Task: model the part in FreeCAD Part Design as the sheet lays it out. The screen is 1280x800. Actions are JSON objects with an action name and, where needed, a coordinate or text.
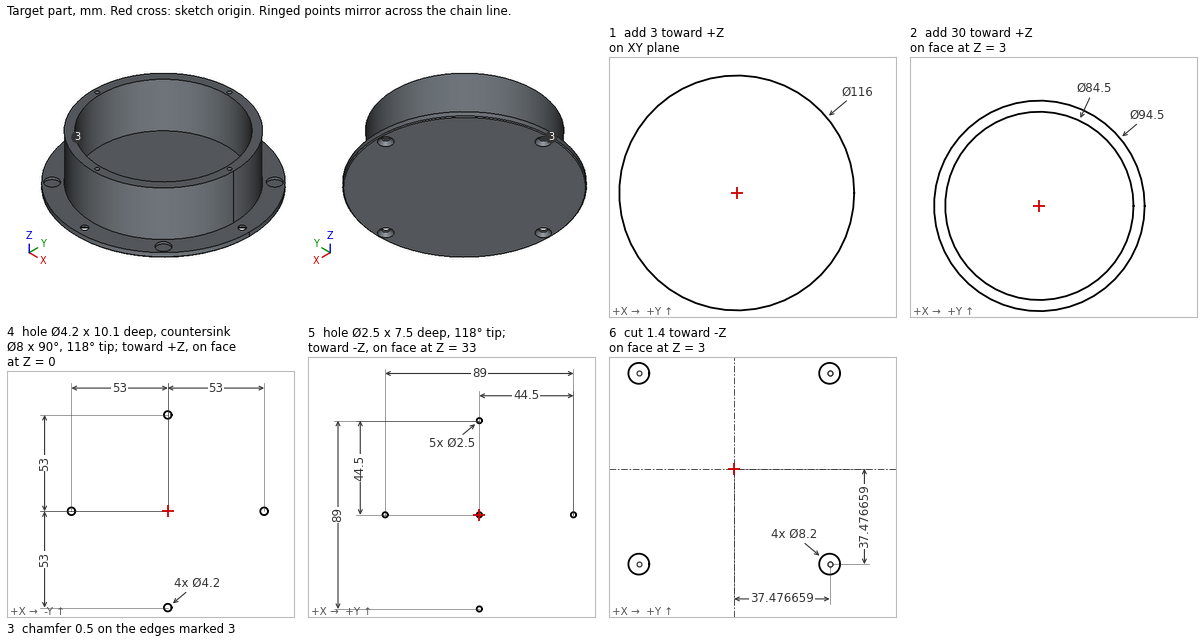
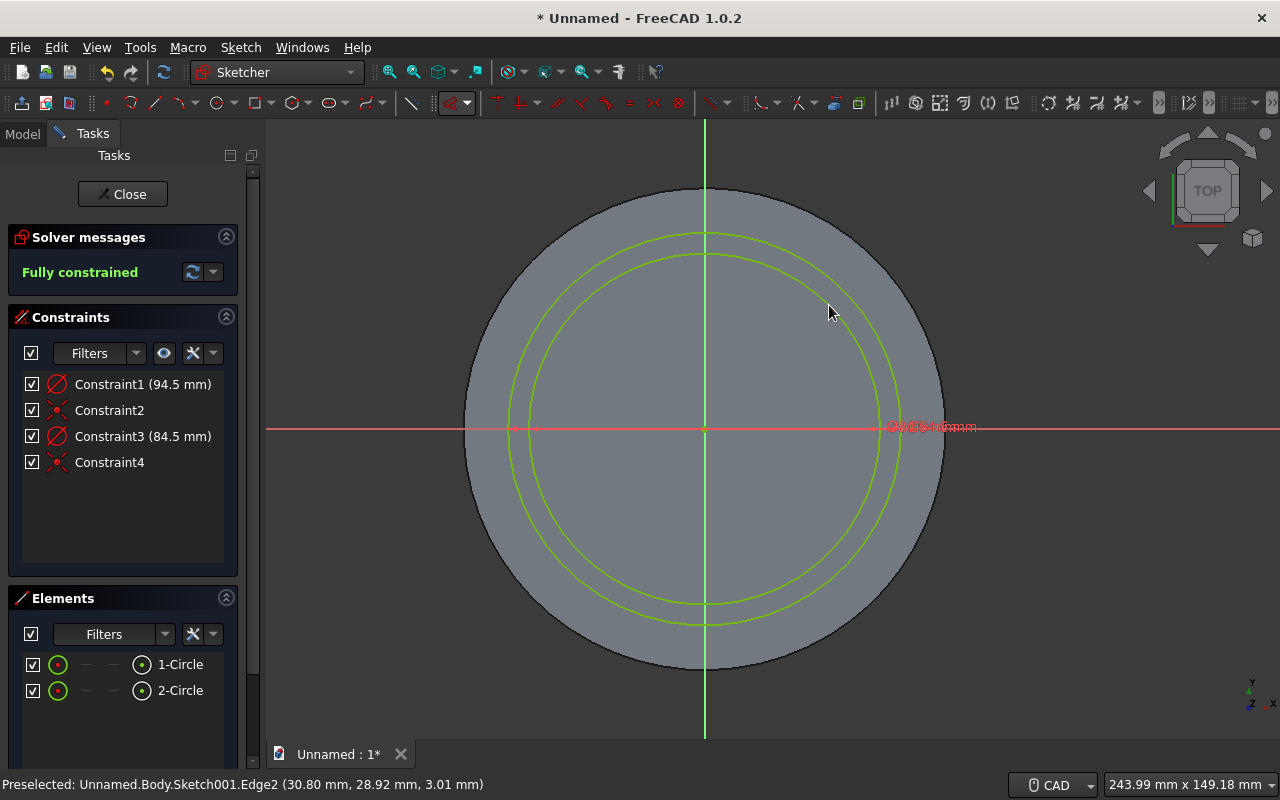
{"action": "left_click", "coordinate": [123, 194]}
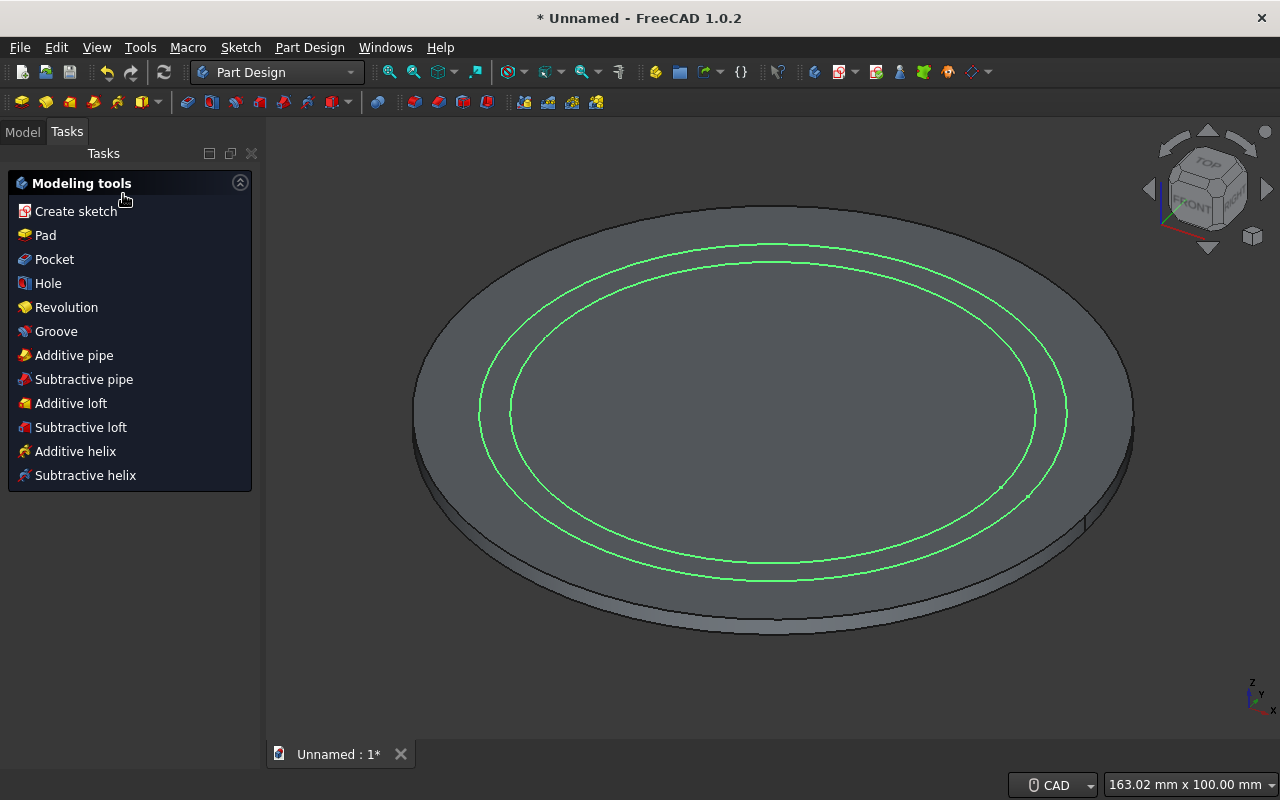
{"action": "left_click", "coordinate": [22, 102]}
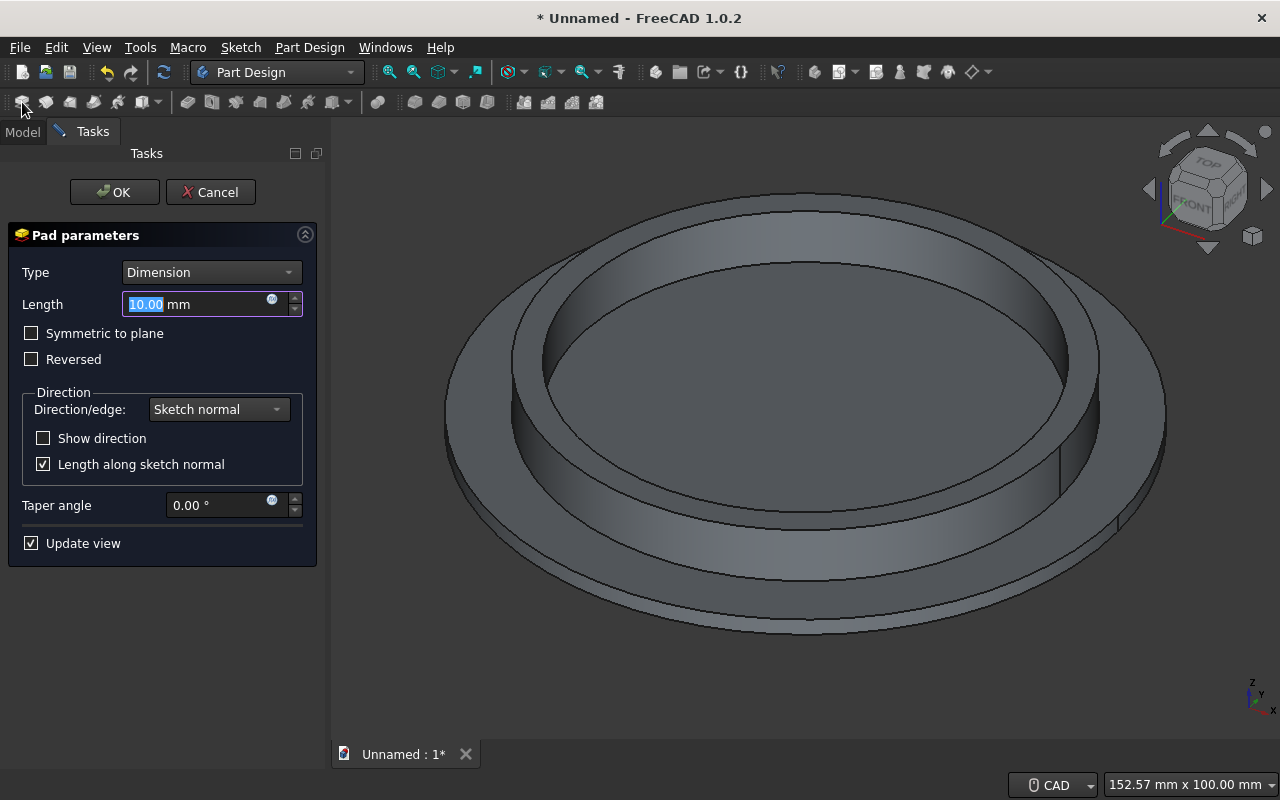
{"action": "type", "text": "30"}
{"action": "key", "text": "Tab"}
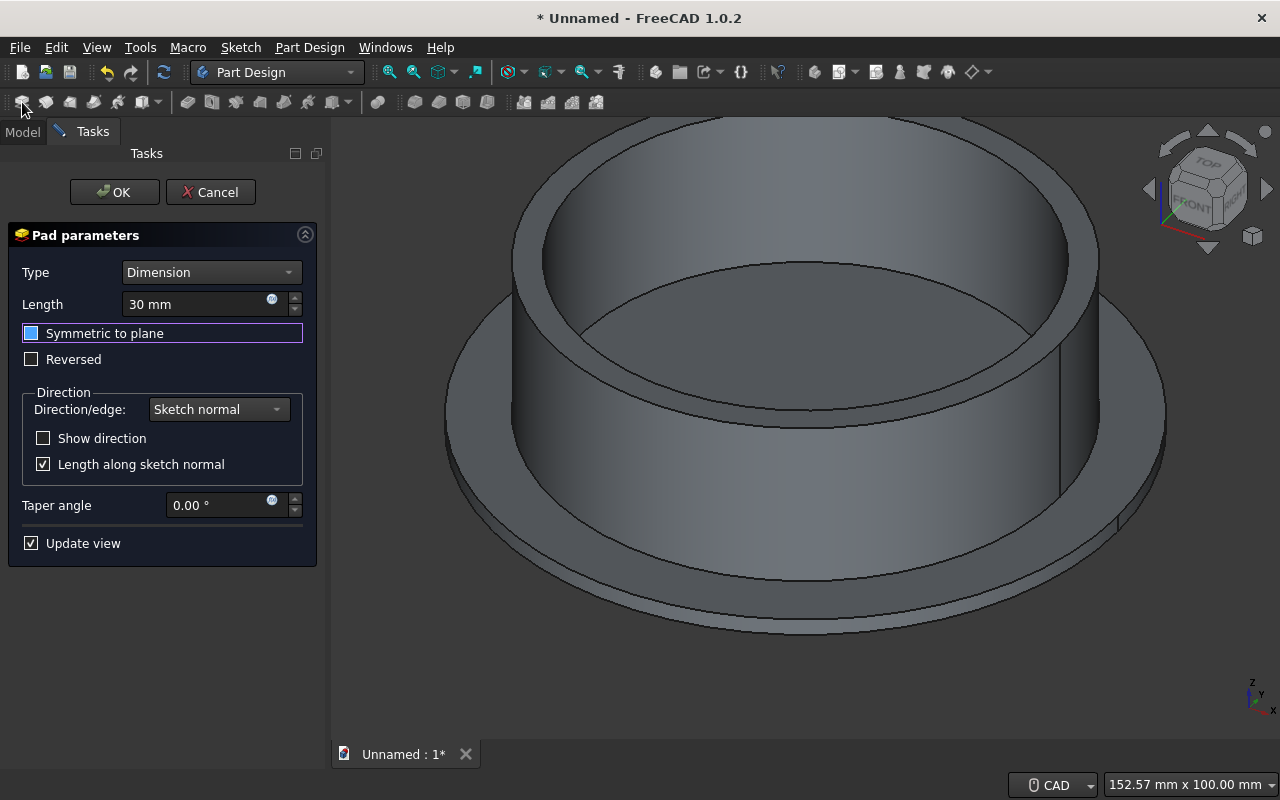
{"action": "left_click", "coordinate": [115, 192]}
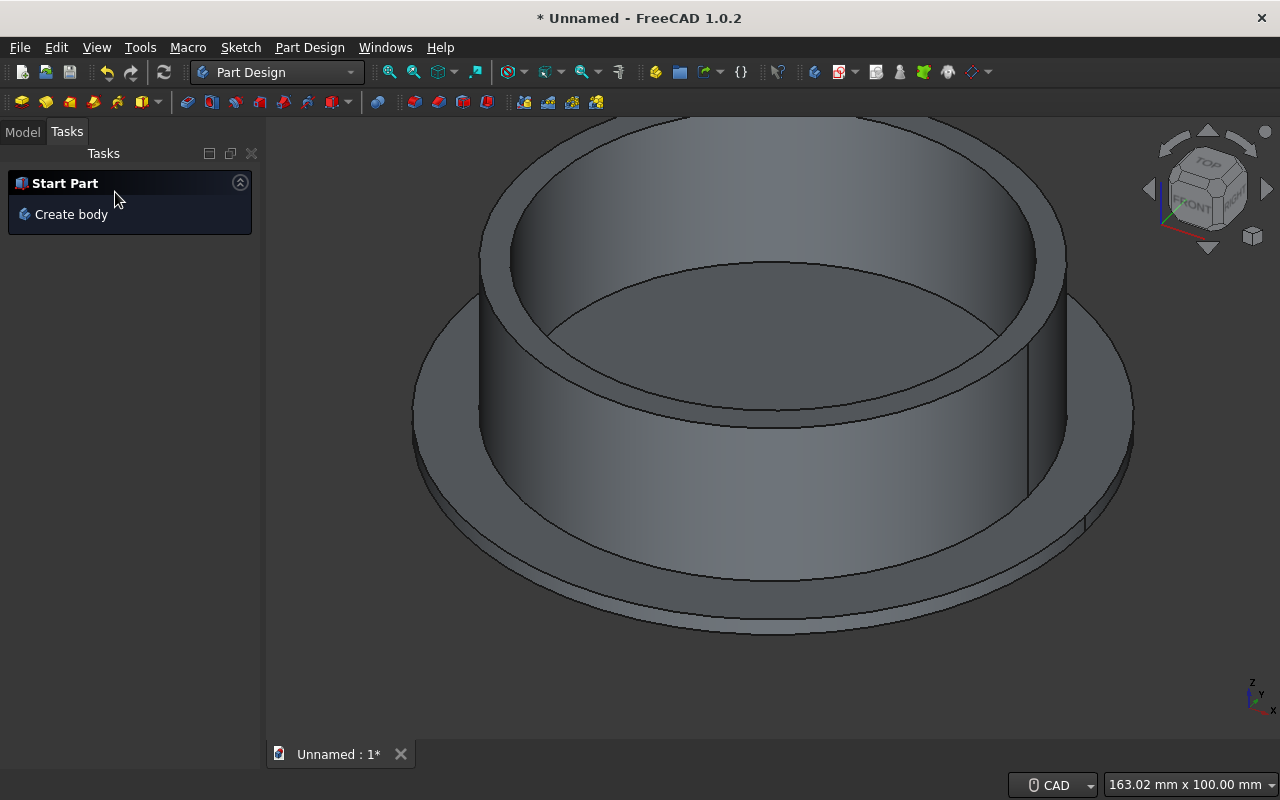
{"action": "left_click", "coordinate": [390, 72]}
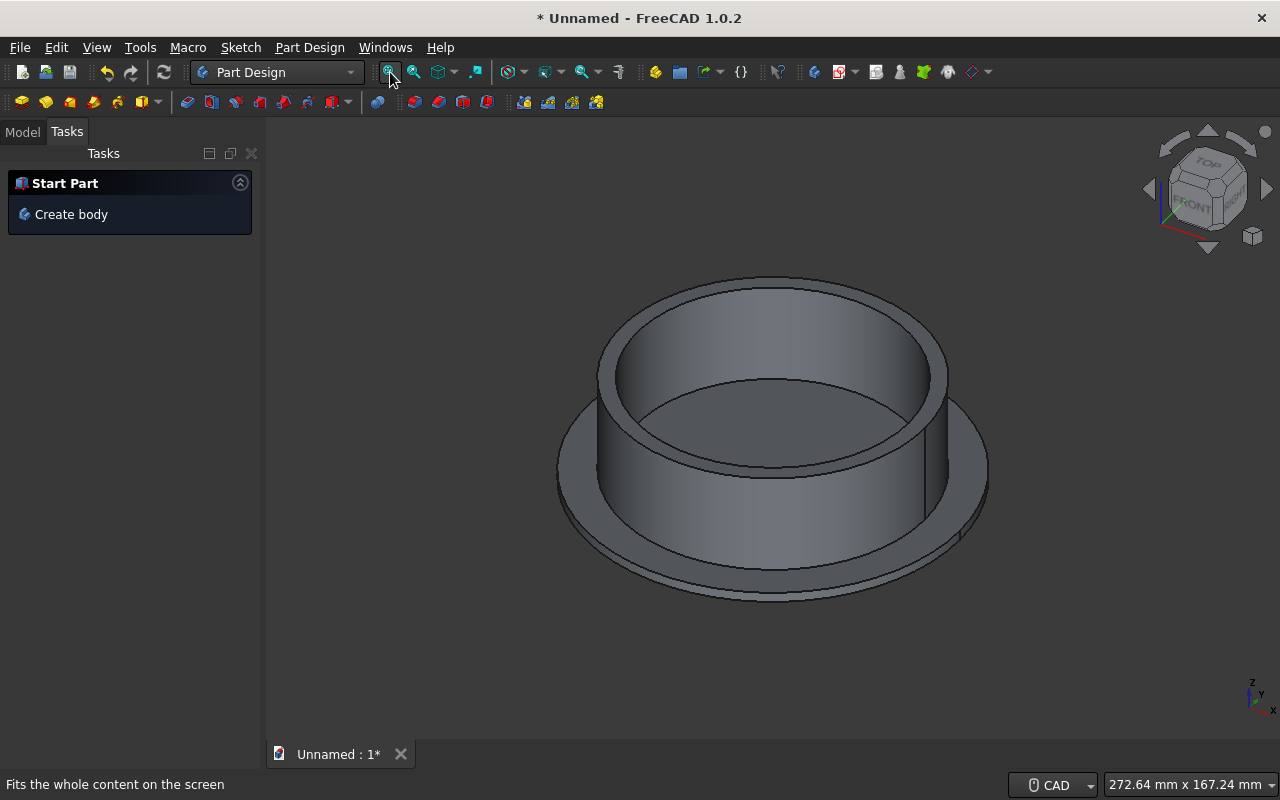
{"action": "left_click", "coordinate": [835, 596]}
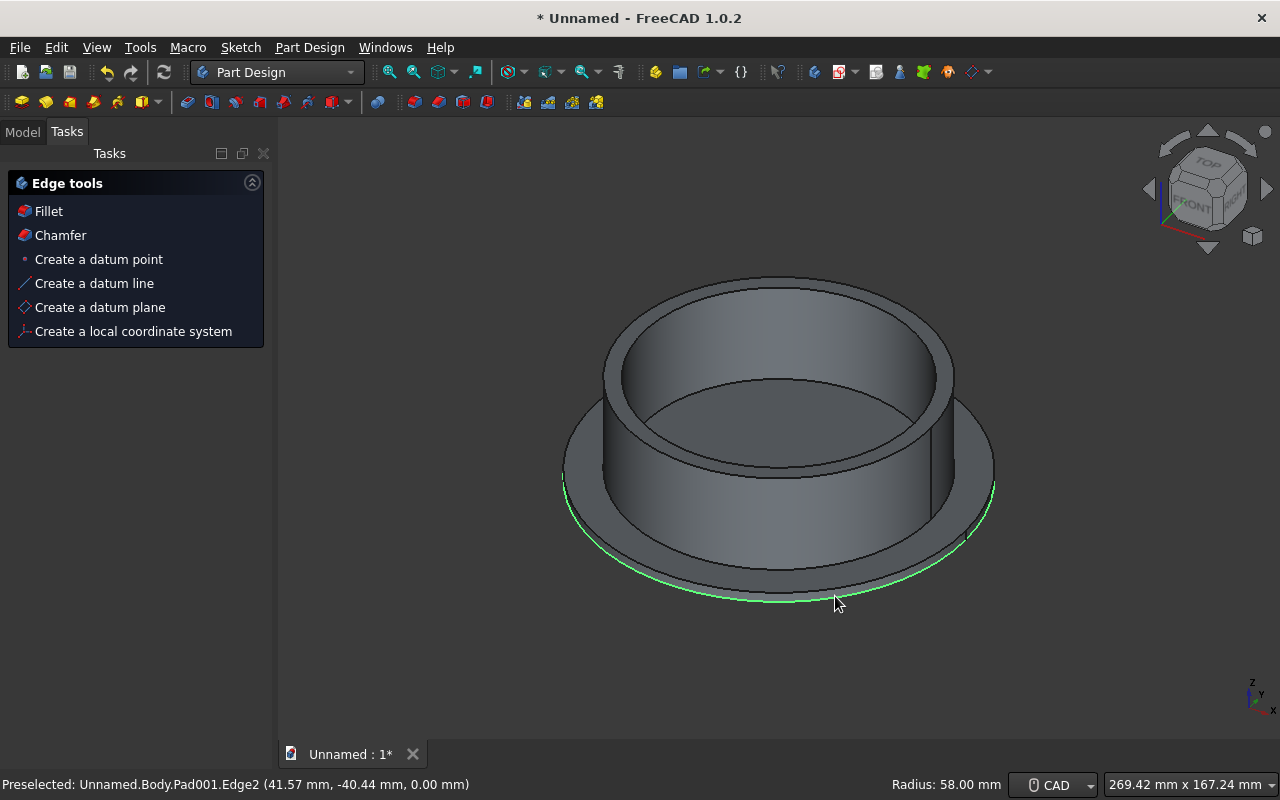
{"action": "left_click", "coordinate": [440, 102]}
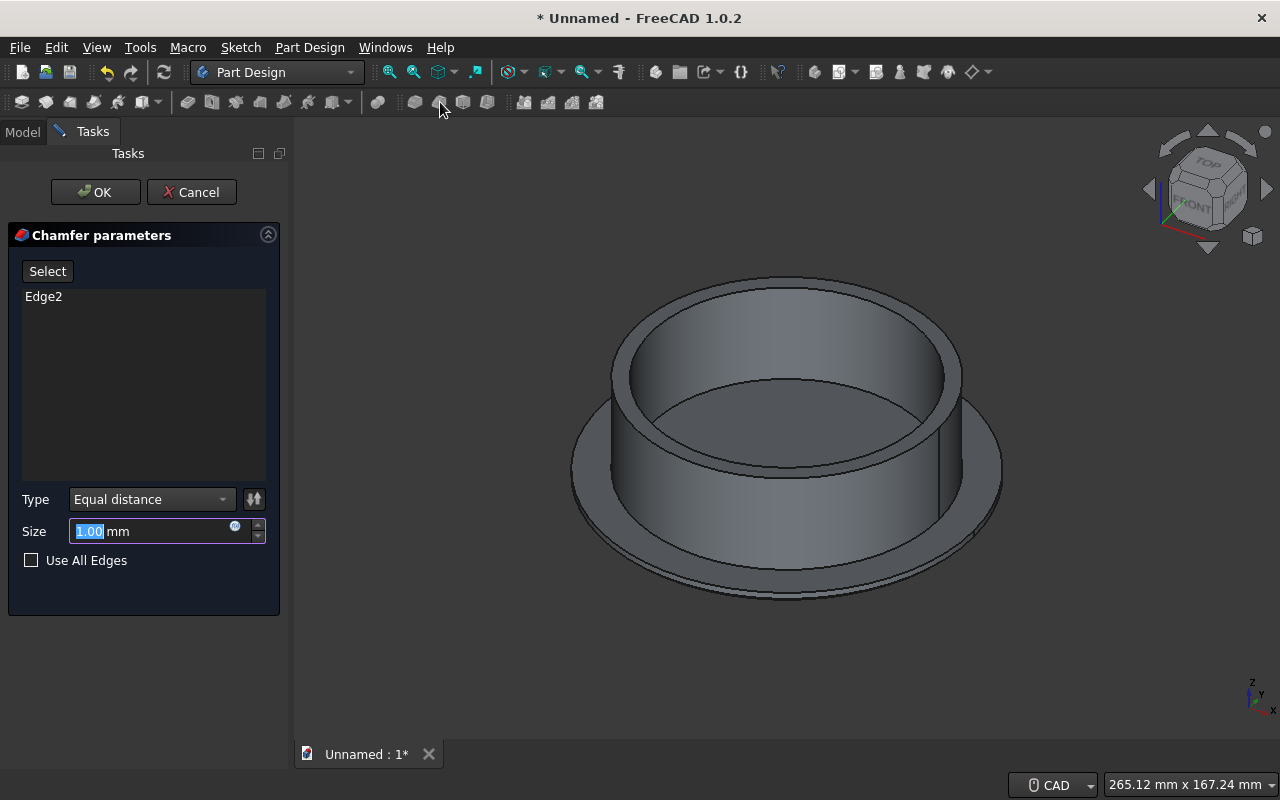
{"action": "type", "text": "0.5"}
{"action": "key", "text": "Tab"}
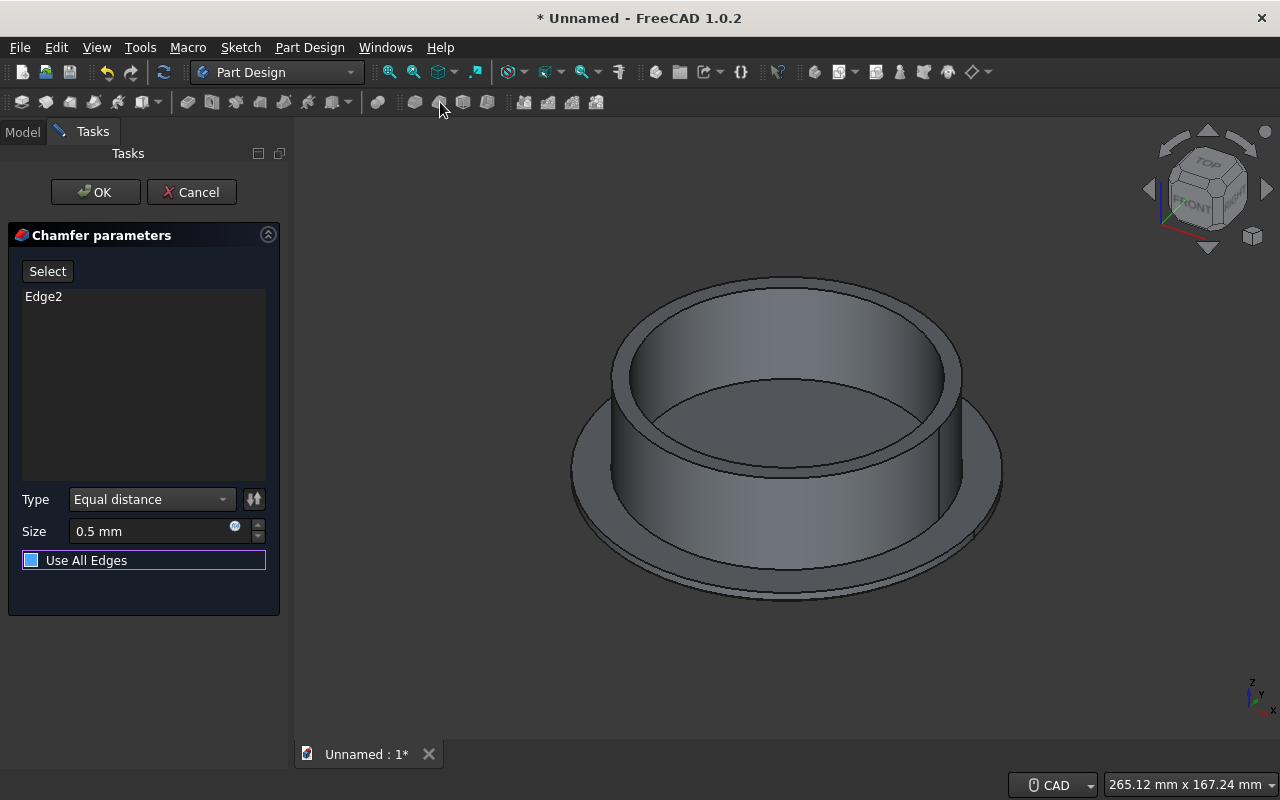
{"action": "left_click", "coordinate": [96, 192]}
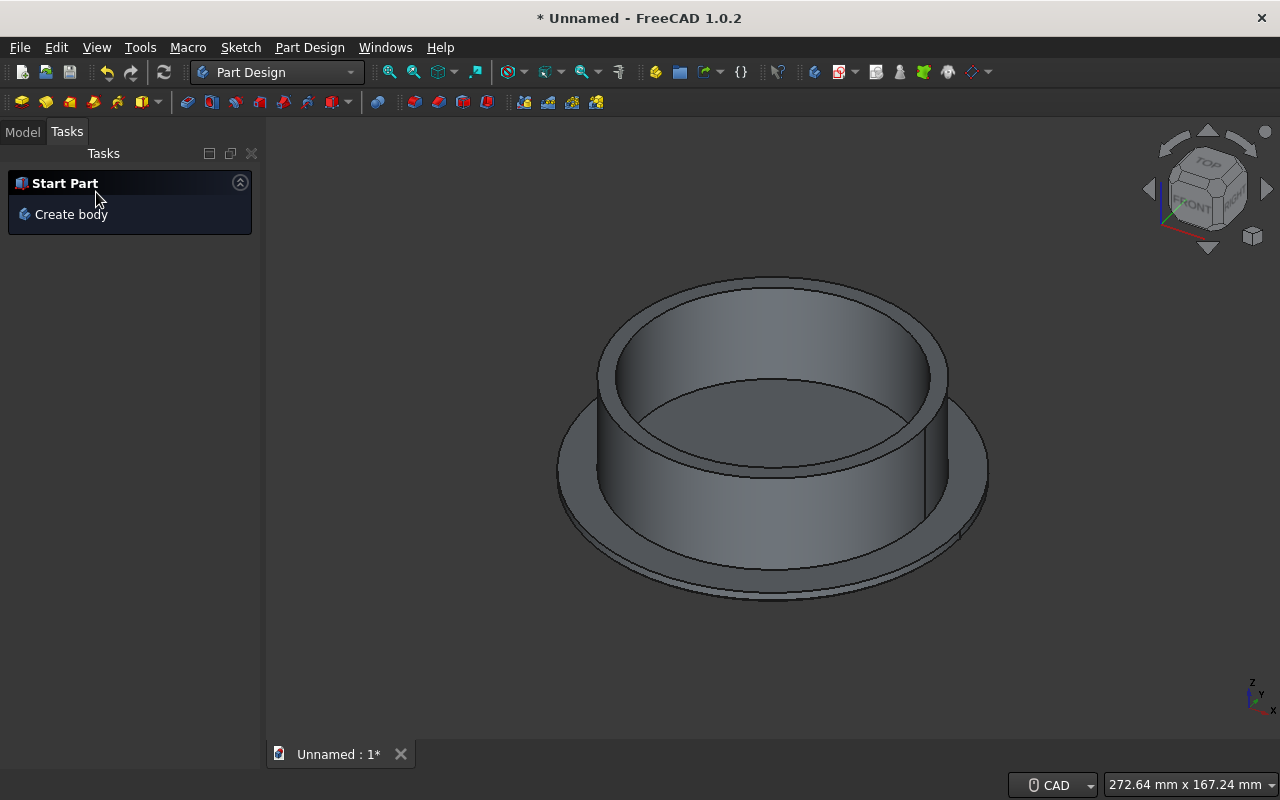
{"action": "key", "text": "5"}